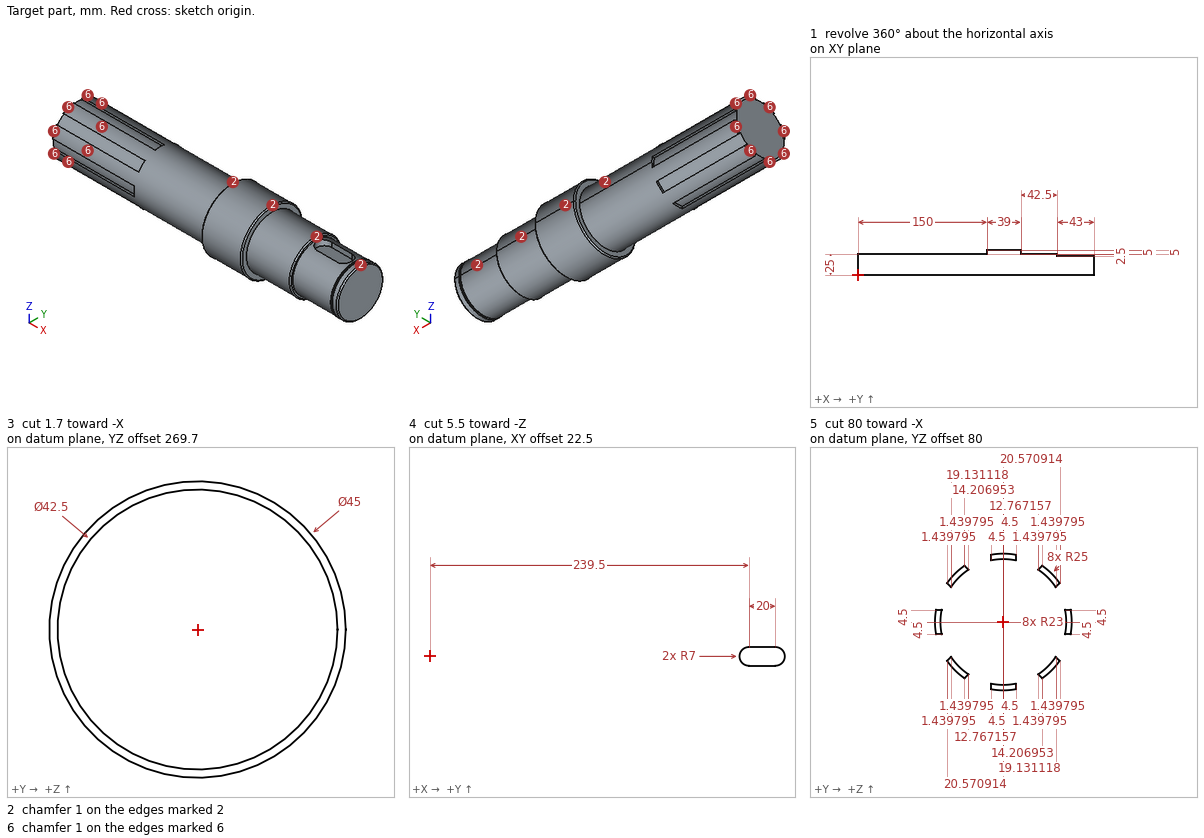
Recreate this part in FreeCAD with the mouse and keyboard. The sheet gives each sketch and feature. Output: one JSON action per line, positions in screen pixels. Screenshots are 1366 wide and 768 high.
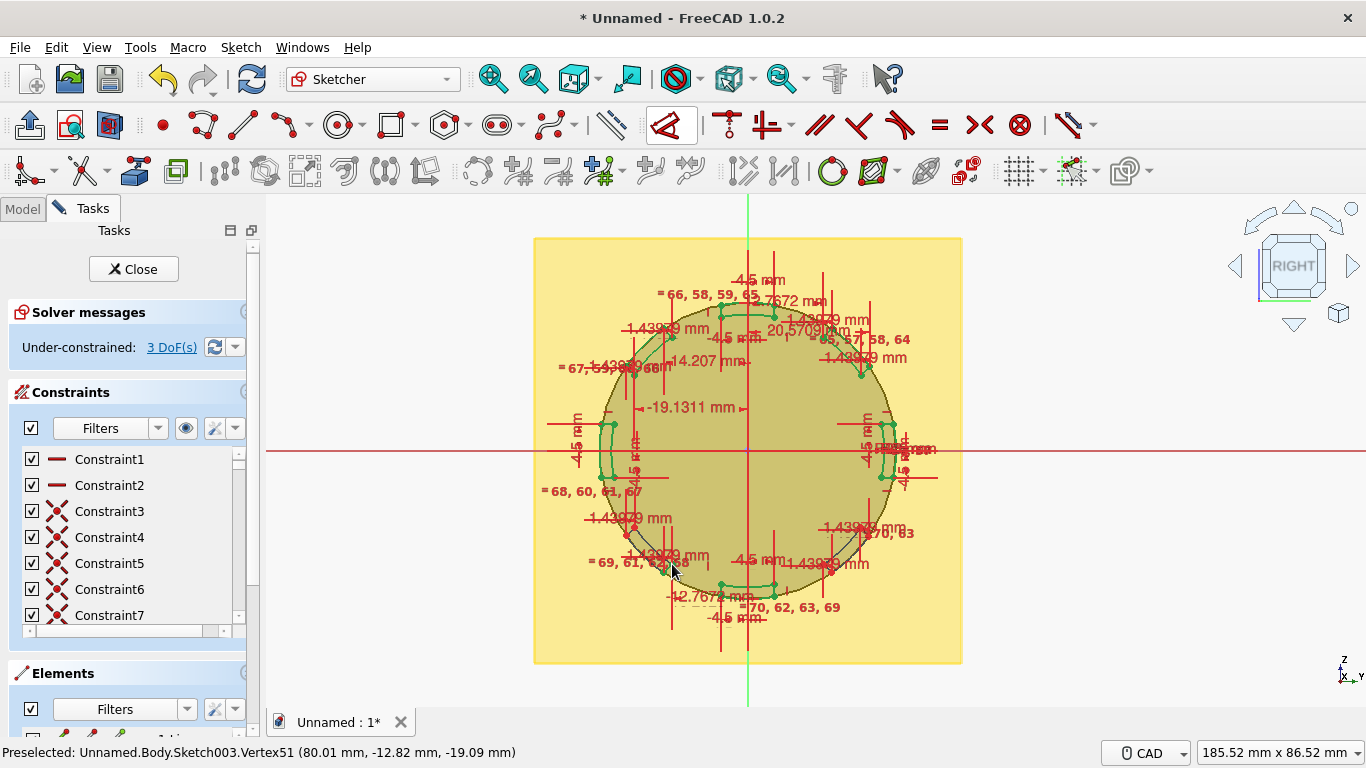
{"action": "left_click", "coordinate": [626, 536]}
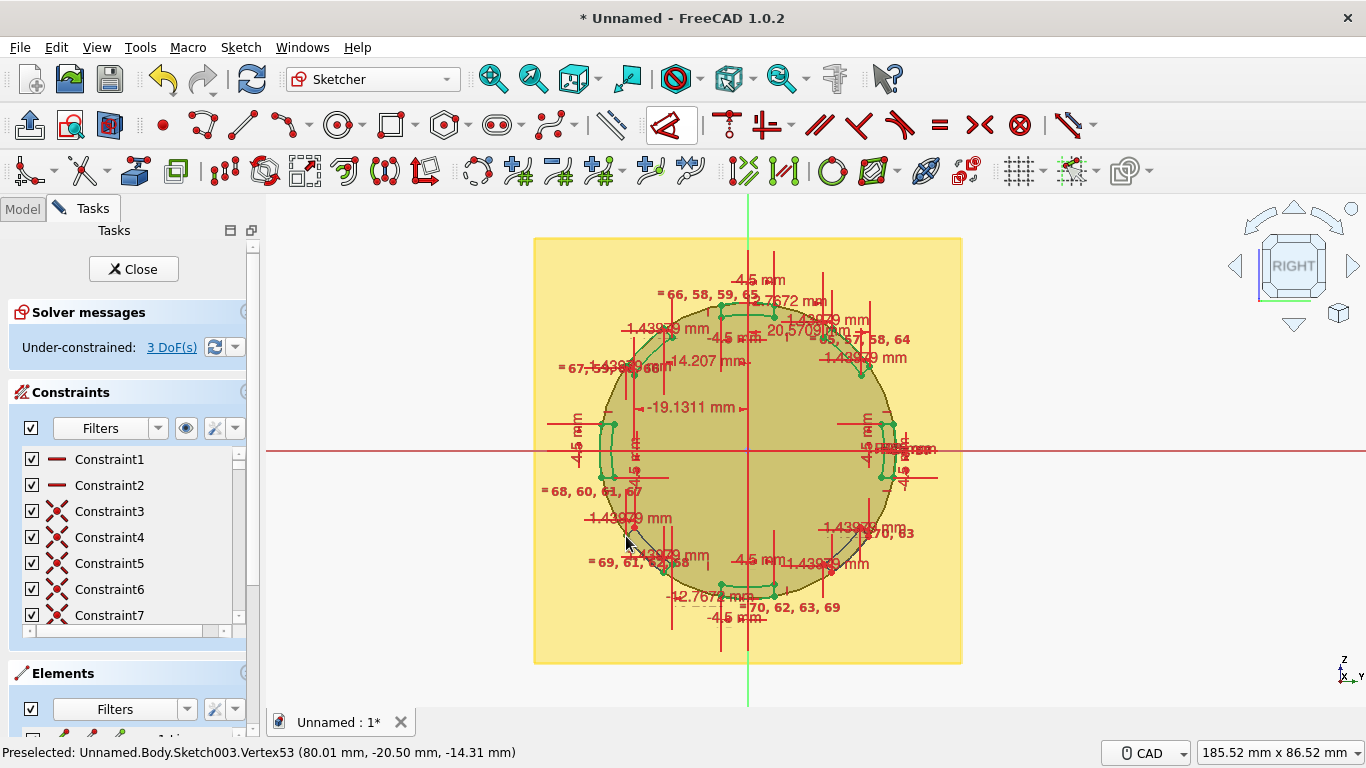
{"action": "key", "text": "l"}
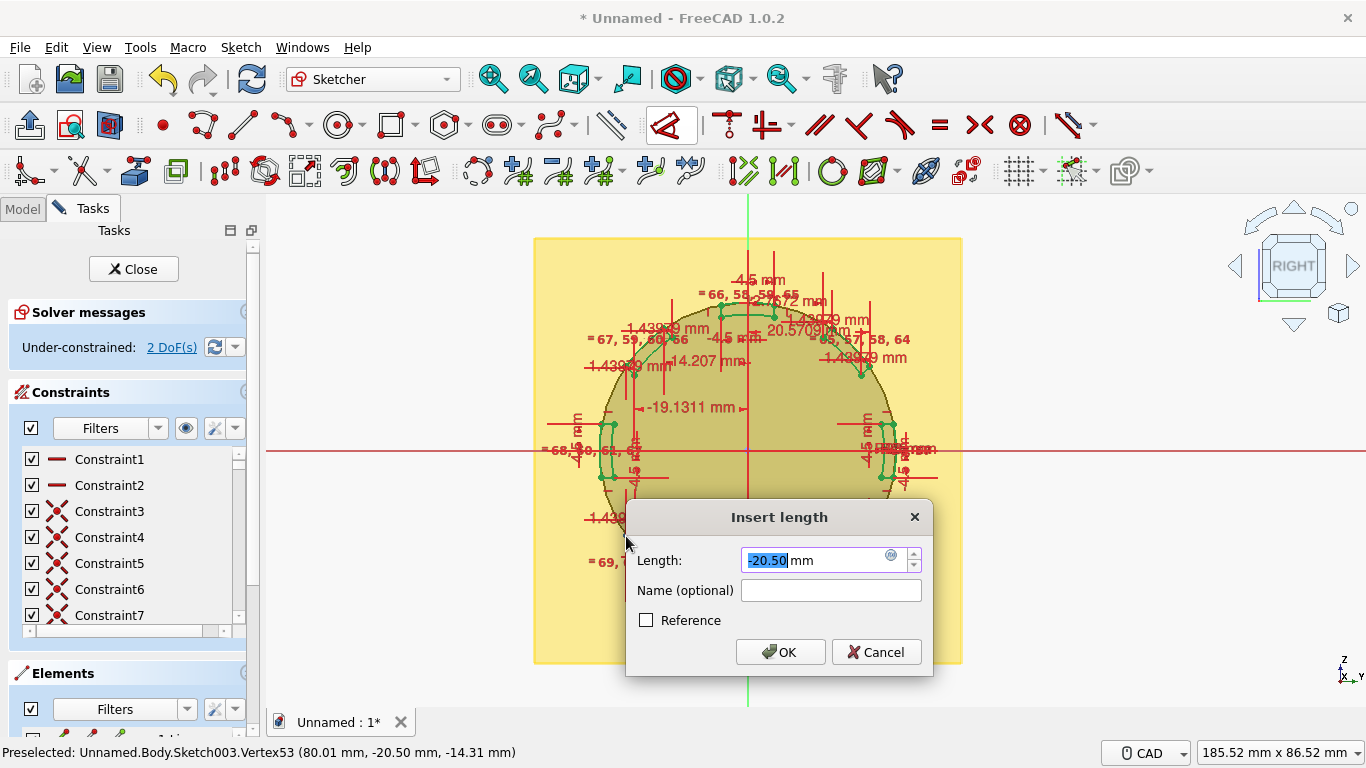
{"action": "type", "text": "-20.570914"}
{"action": "key", "text": "Return"}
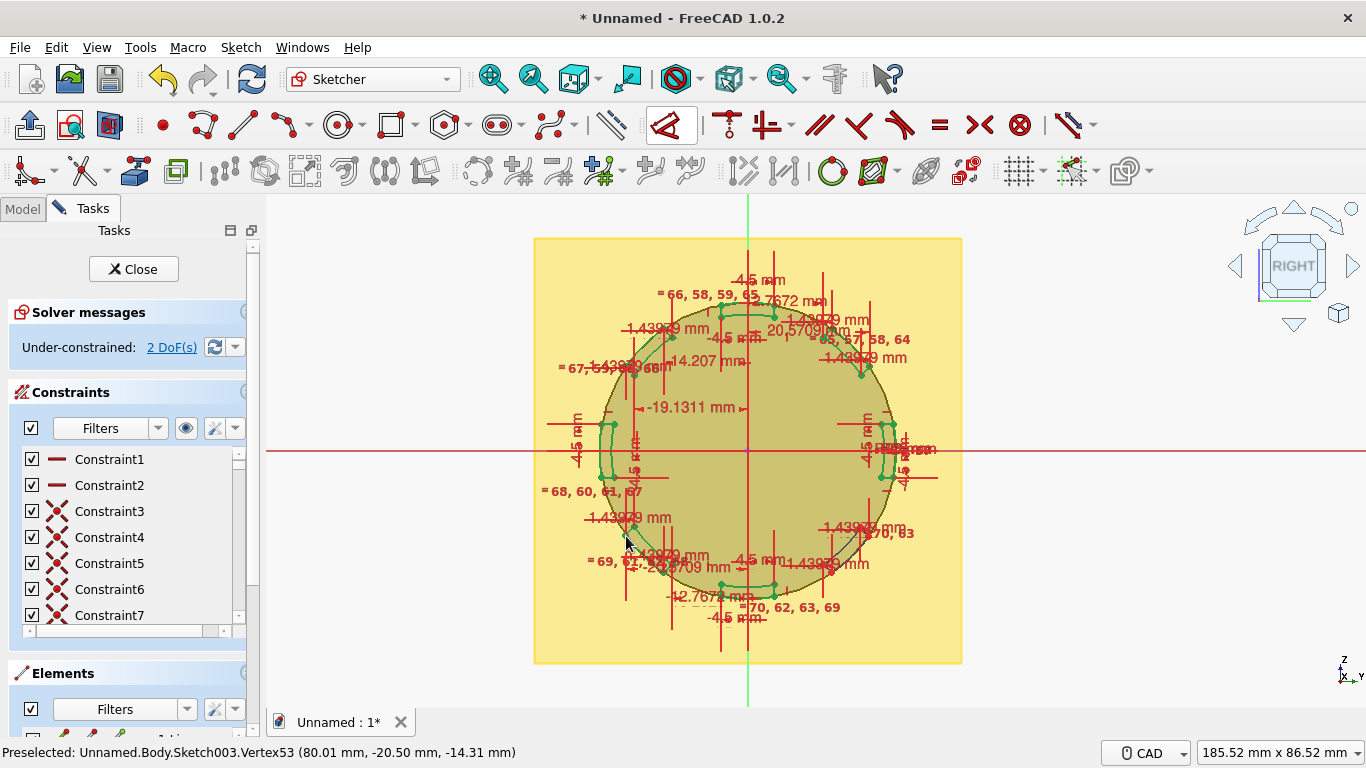
{"action": "left_click", "coordinate": [860, 528]}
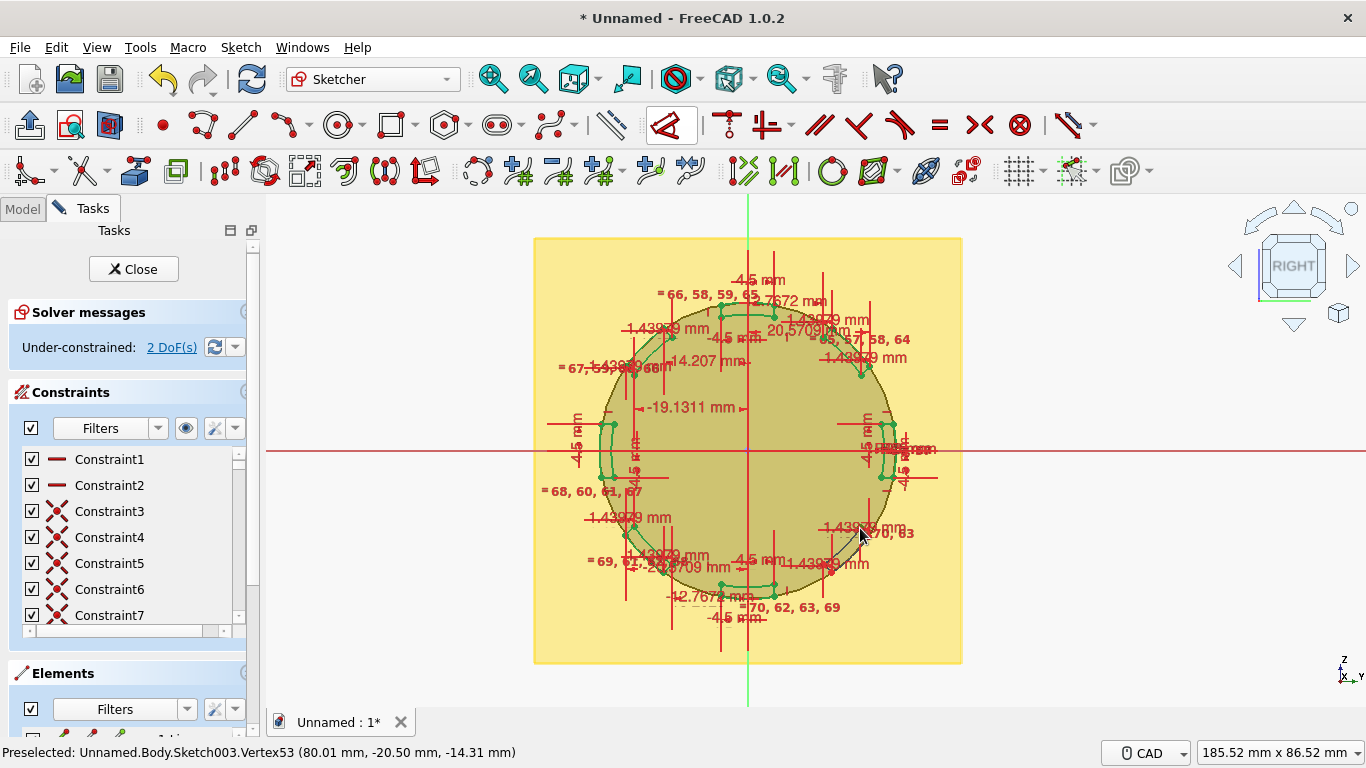
{"action": "key", "text": "l"}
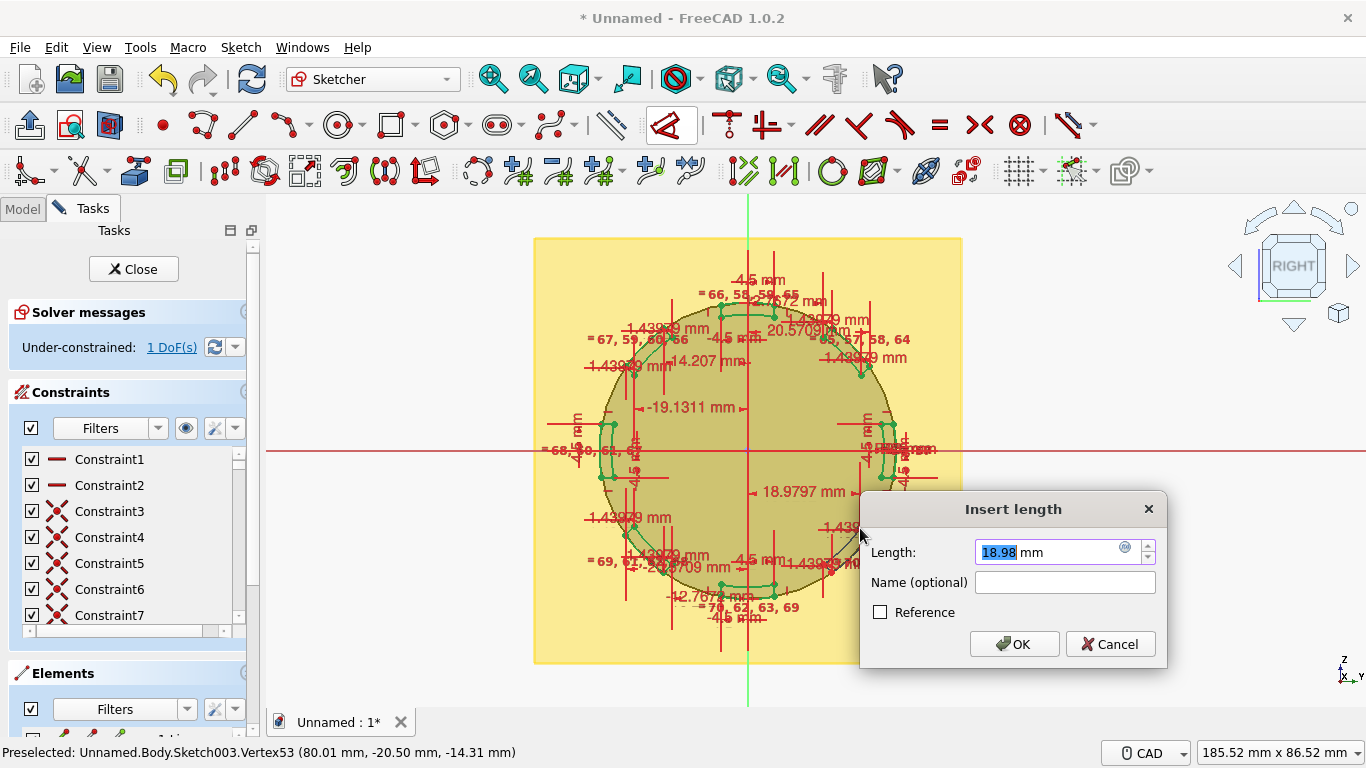
{"action": "type", "text": "19.131118"}
{"action": "key", "text": "Return"}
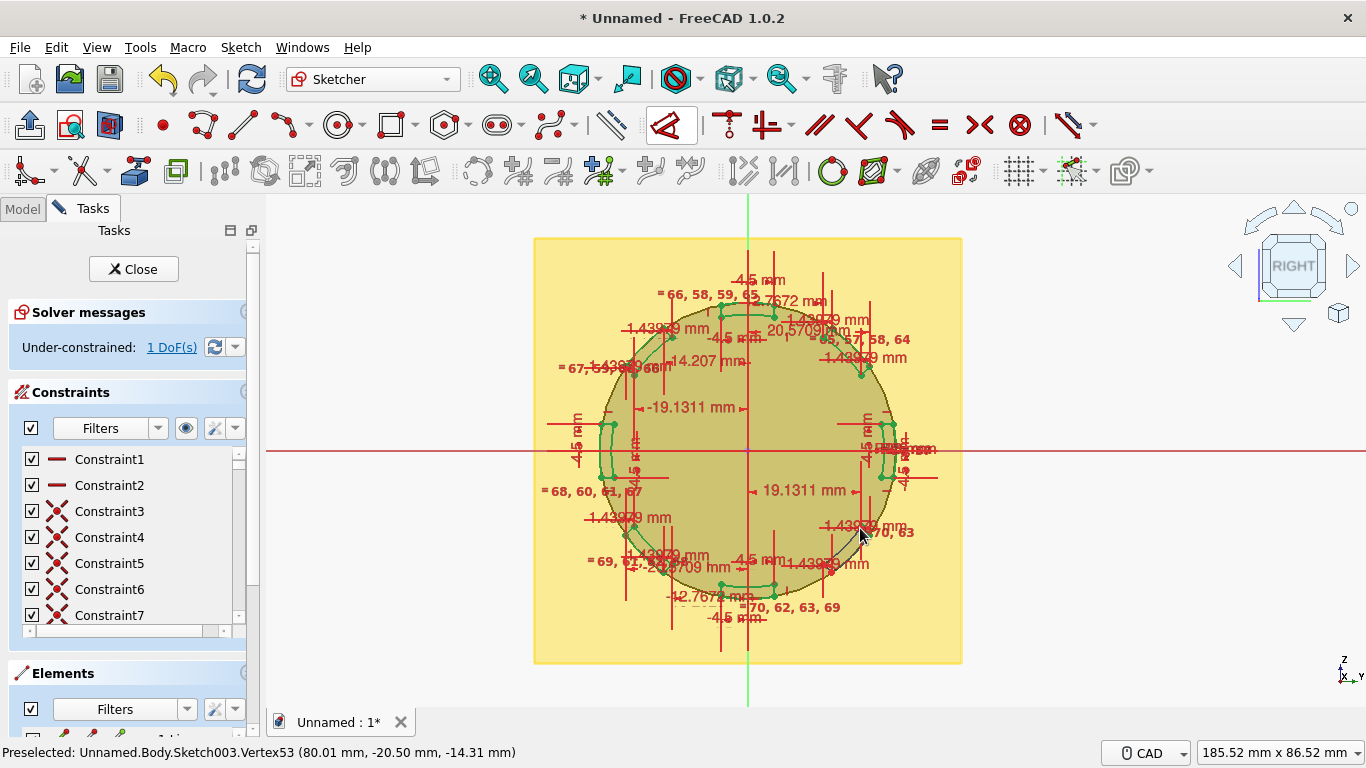
{"action": "left_click", "coordinate": [832, 573]}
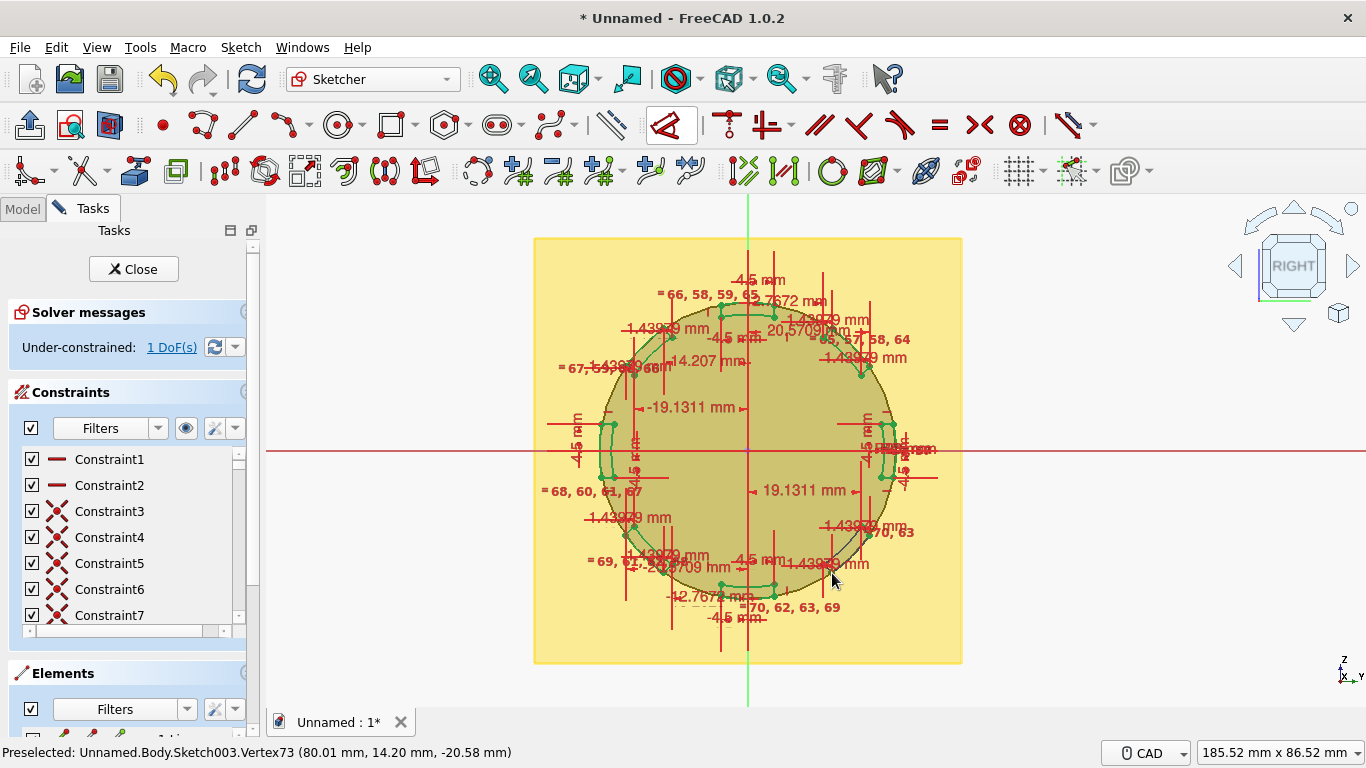
{"action": "left_click", "coordinate": [692, 126]}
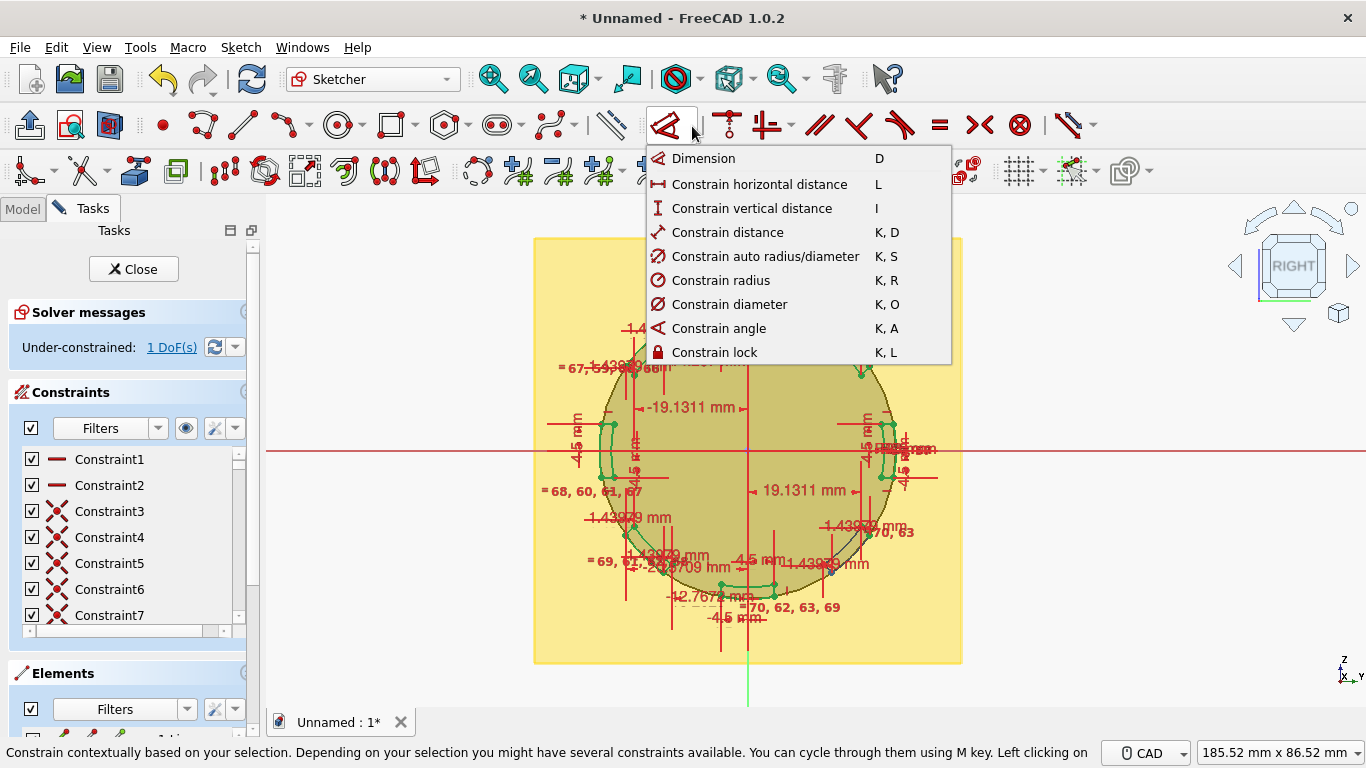
{"action": "left_click", "coordinate": [799, 184]}